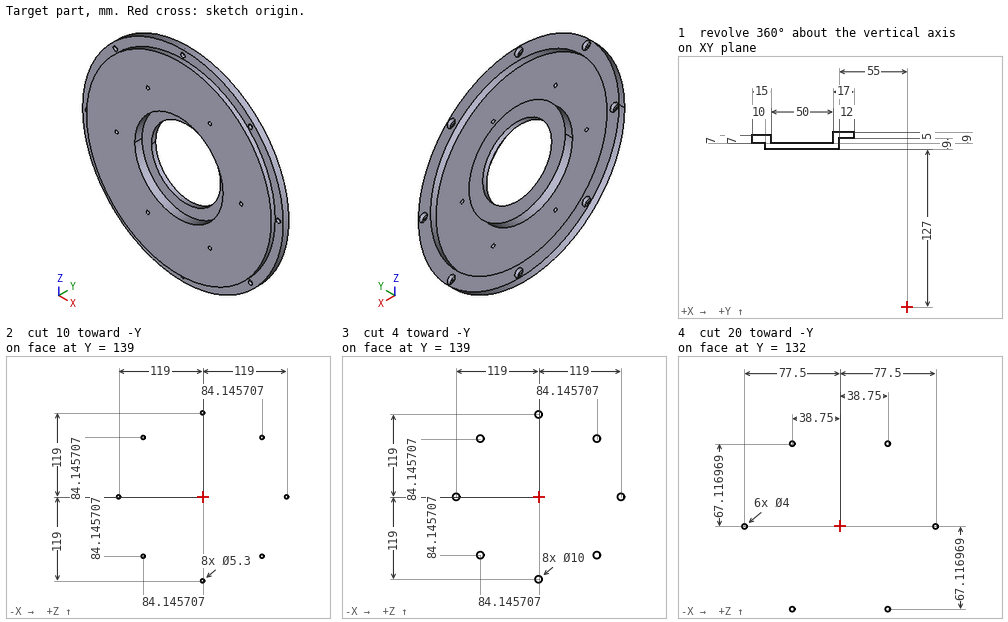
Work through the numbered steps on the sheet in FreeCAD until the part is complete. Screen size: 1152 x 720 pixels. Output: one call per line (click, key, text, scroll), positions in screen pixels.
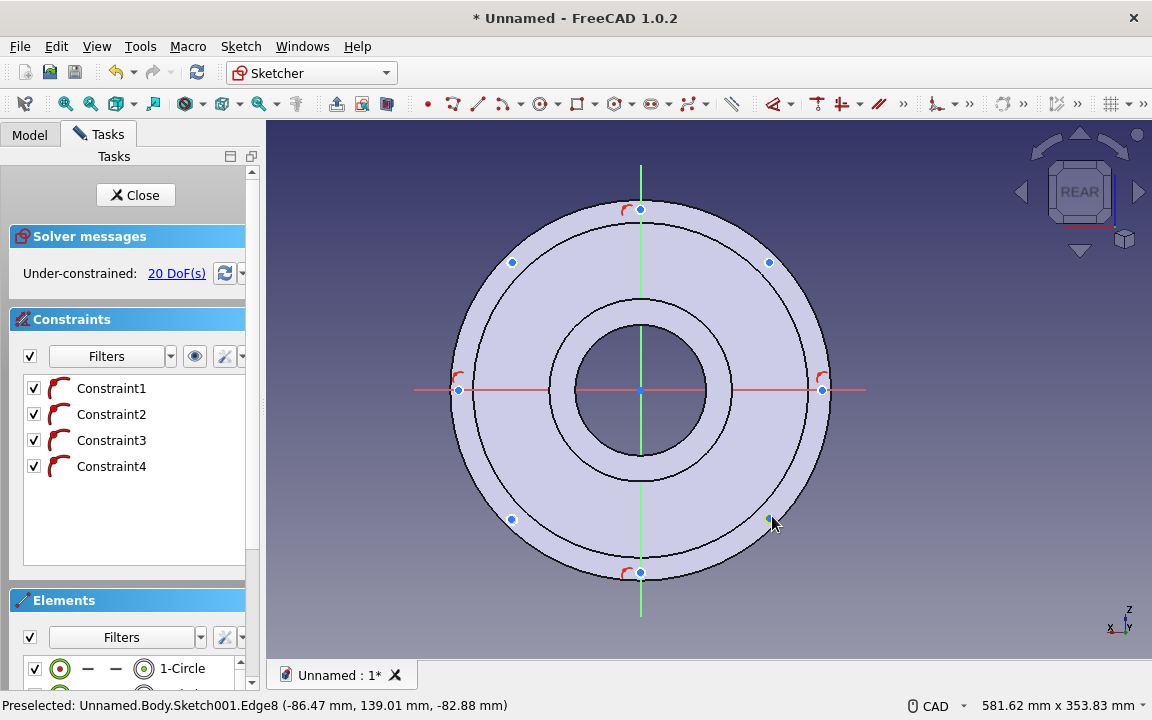
scroll(644, 570, up, 8)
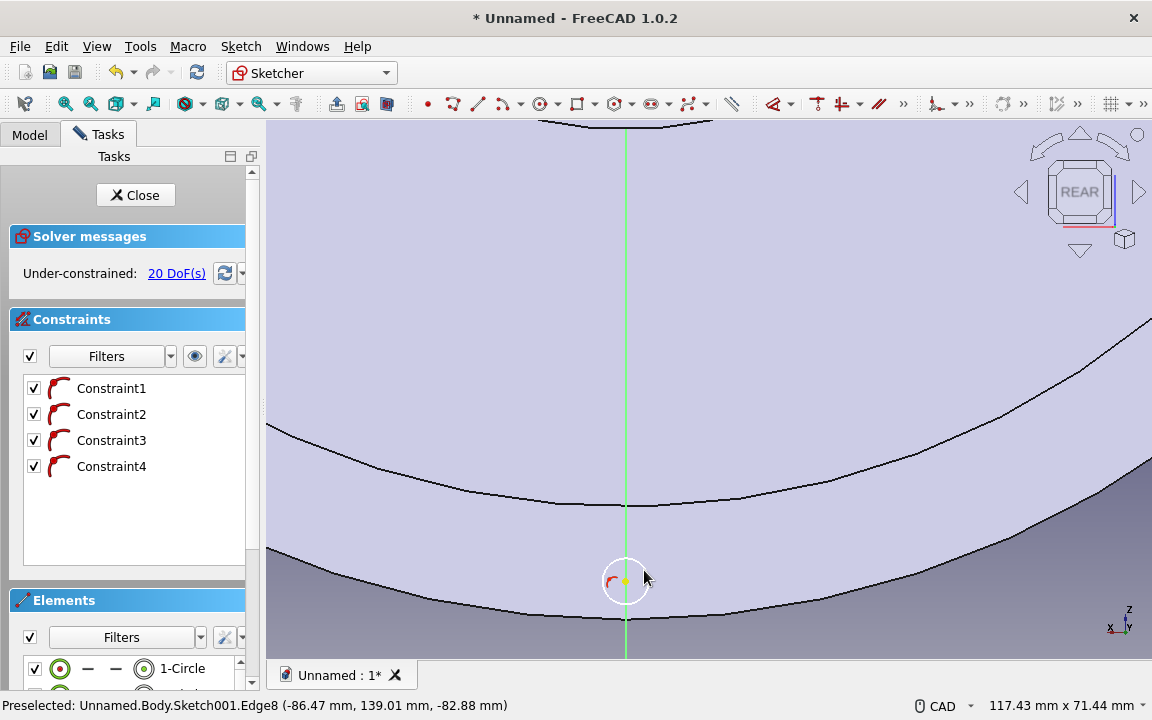
click(642, 565)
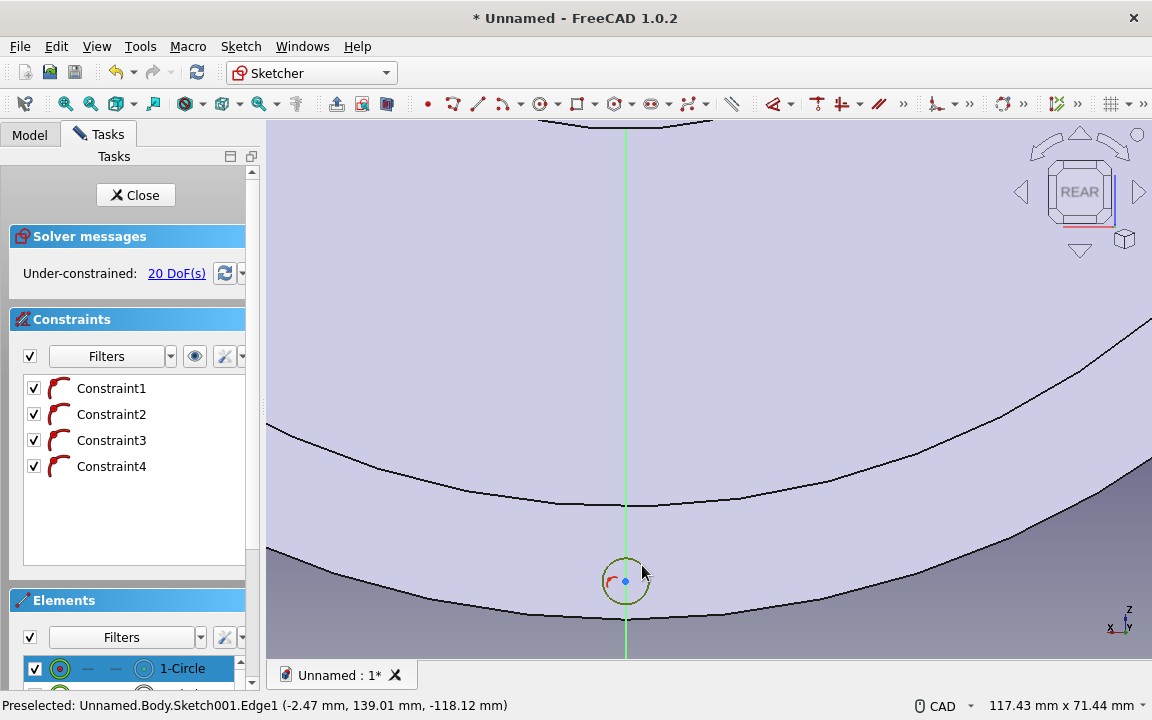
scroll(644, 570, down, 8)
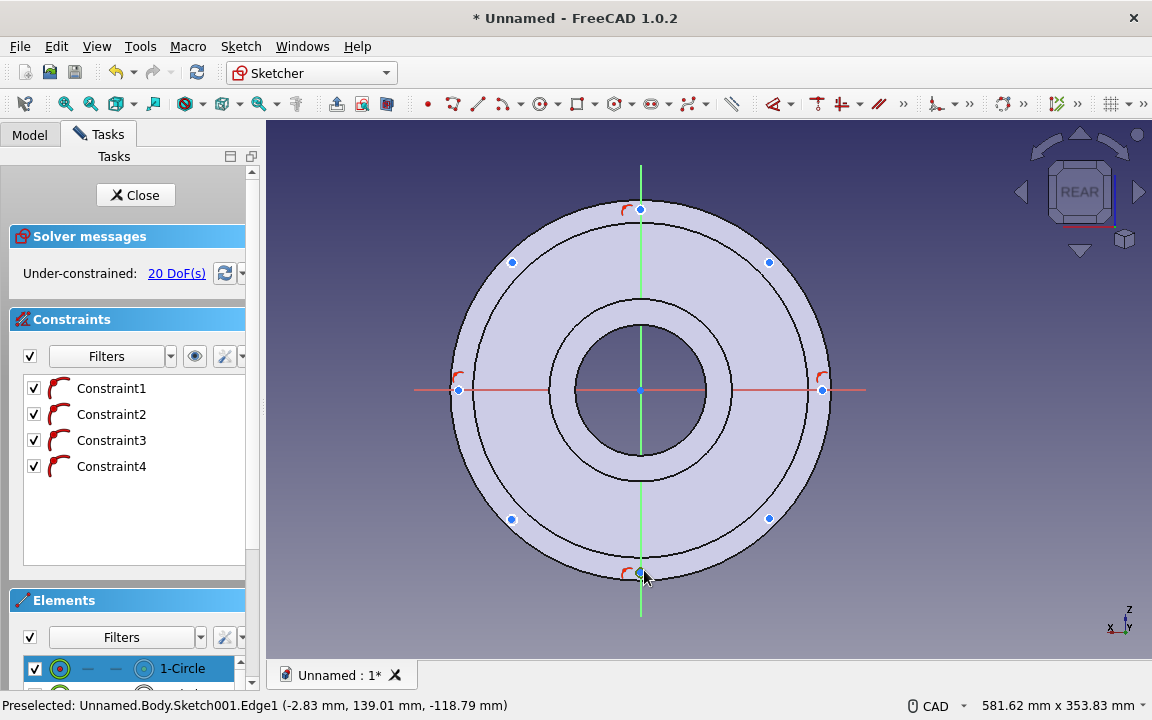
scroll(516, 516, up, 5)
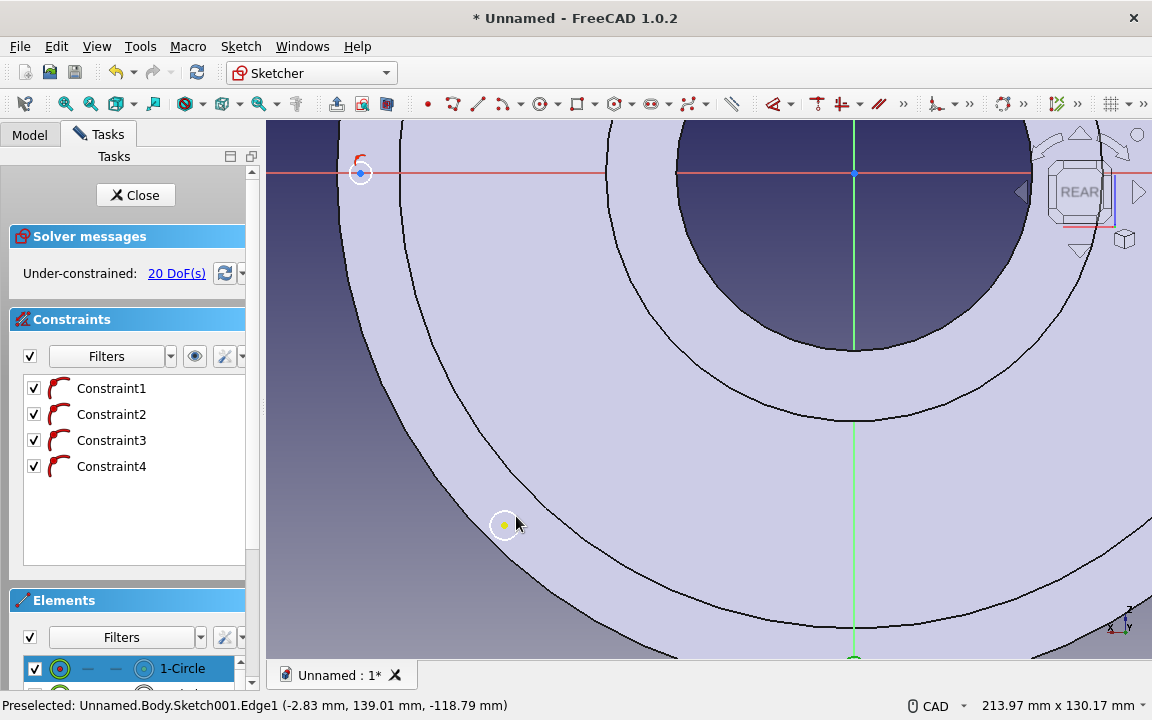
click(515, 515)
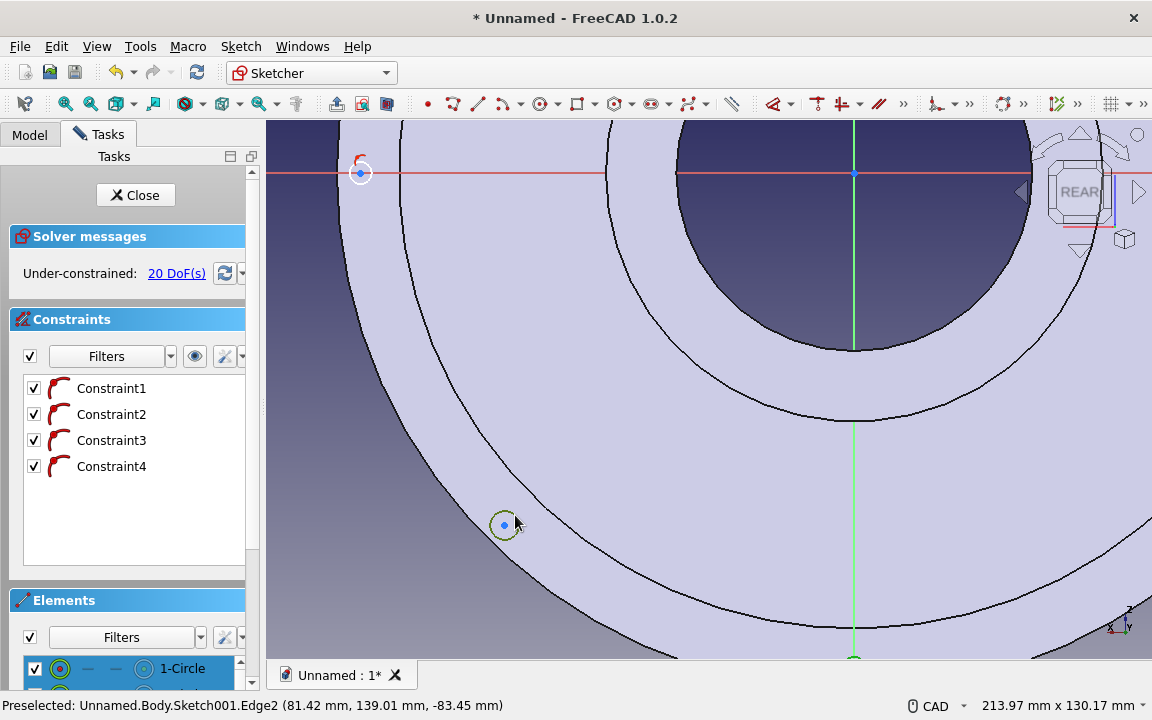
scroll(361, 162, up, 2)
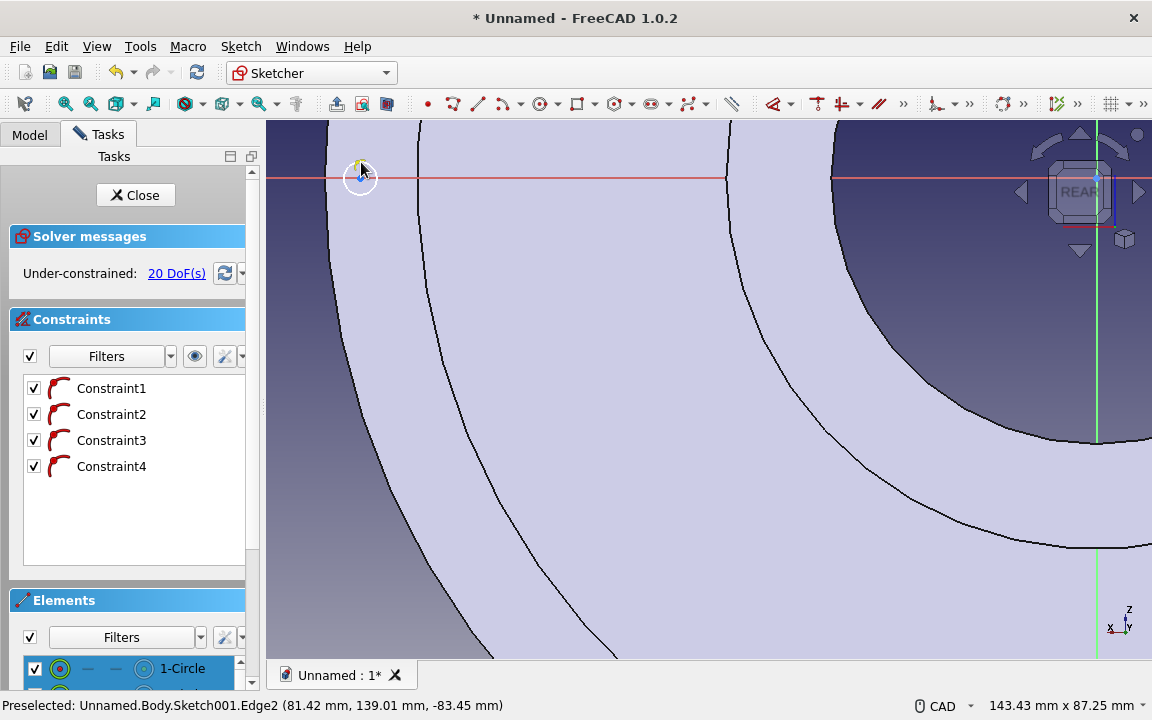
click(344, 178)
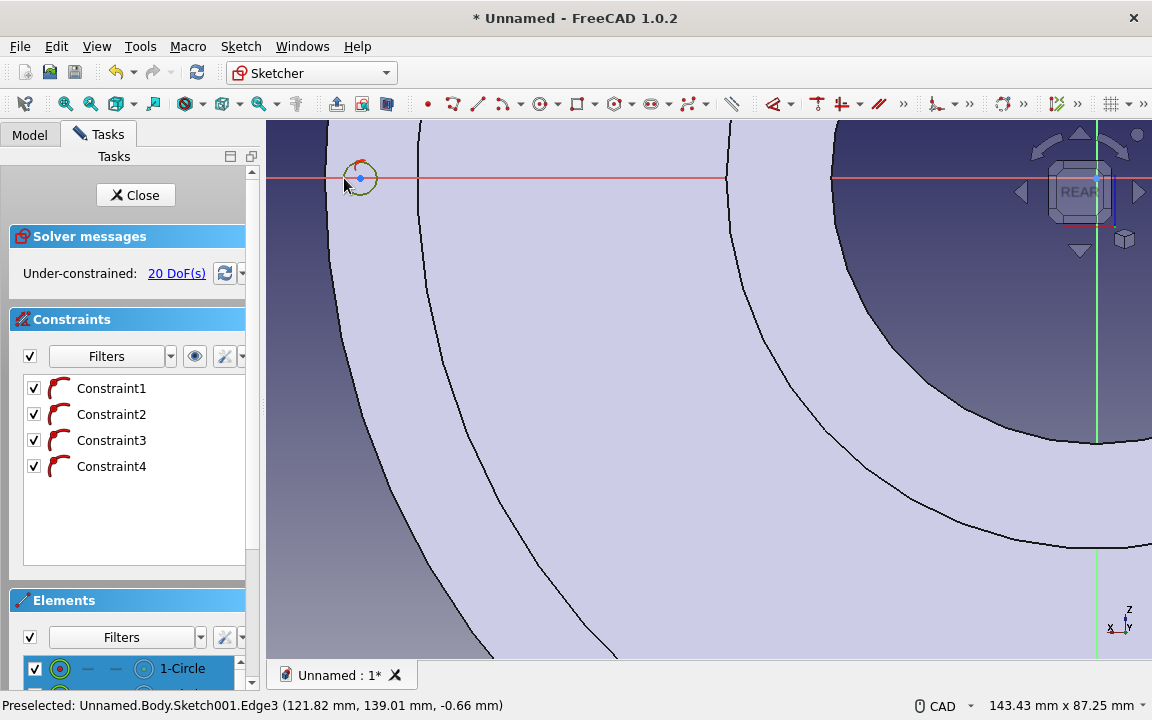
scroll(491, 459, down, 7)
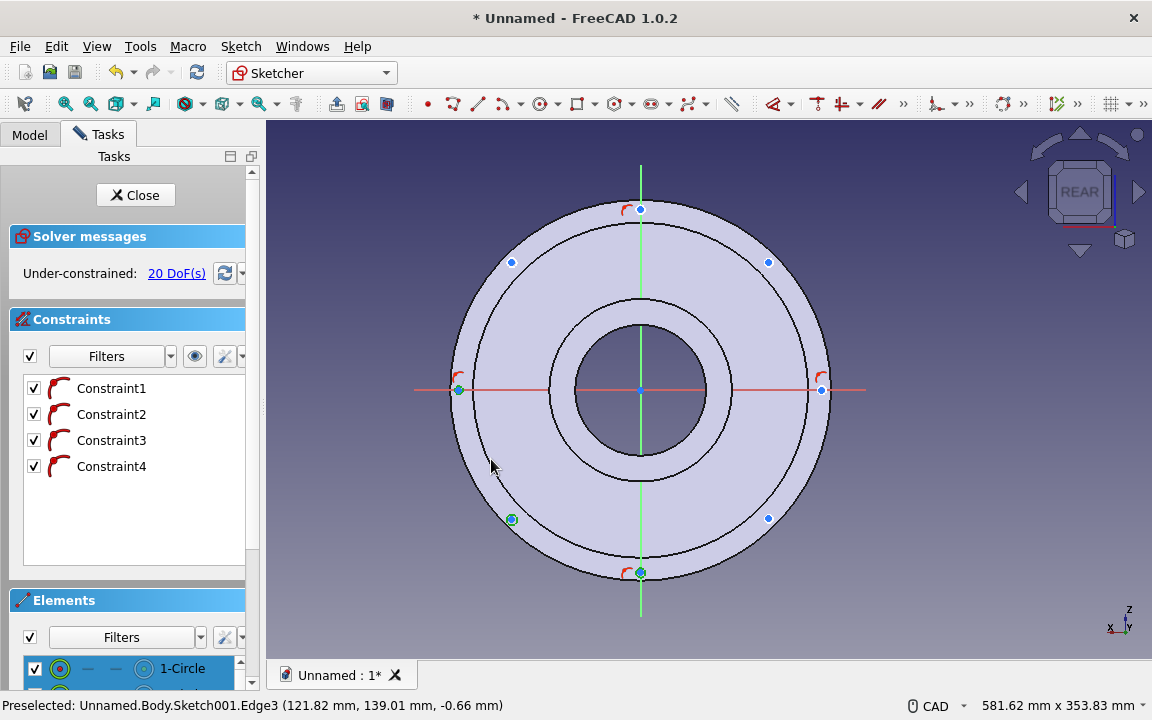
scroll(515, 260, up, 6)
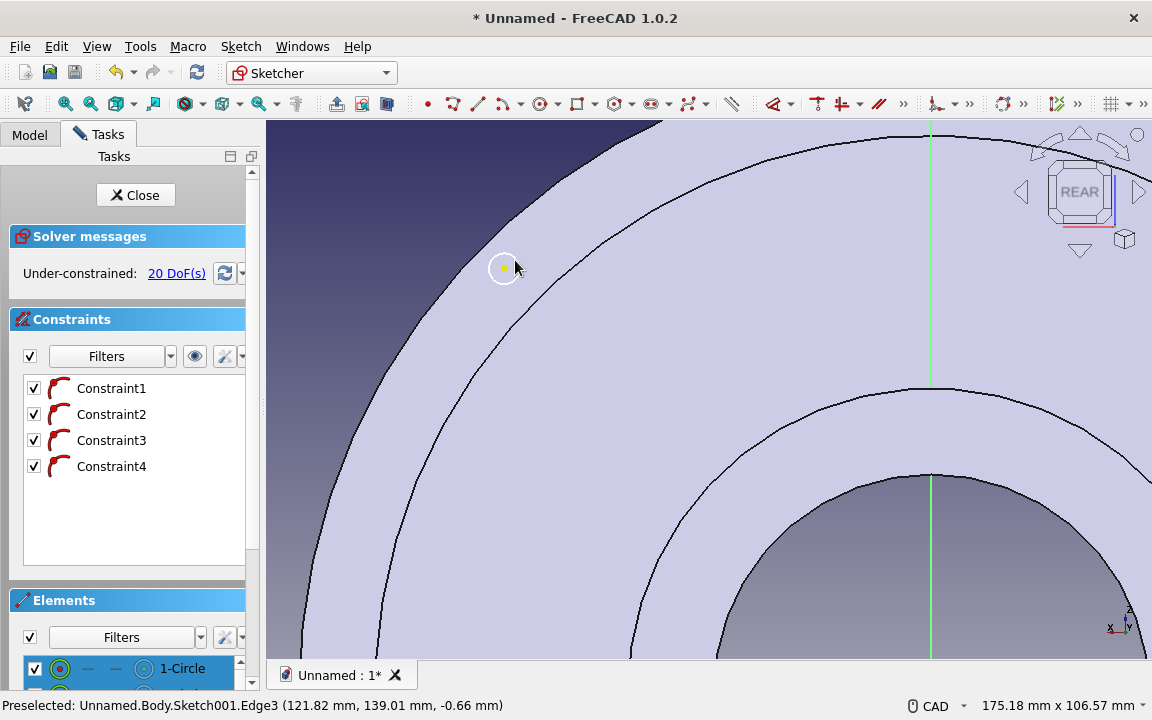
click(515, 258)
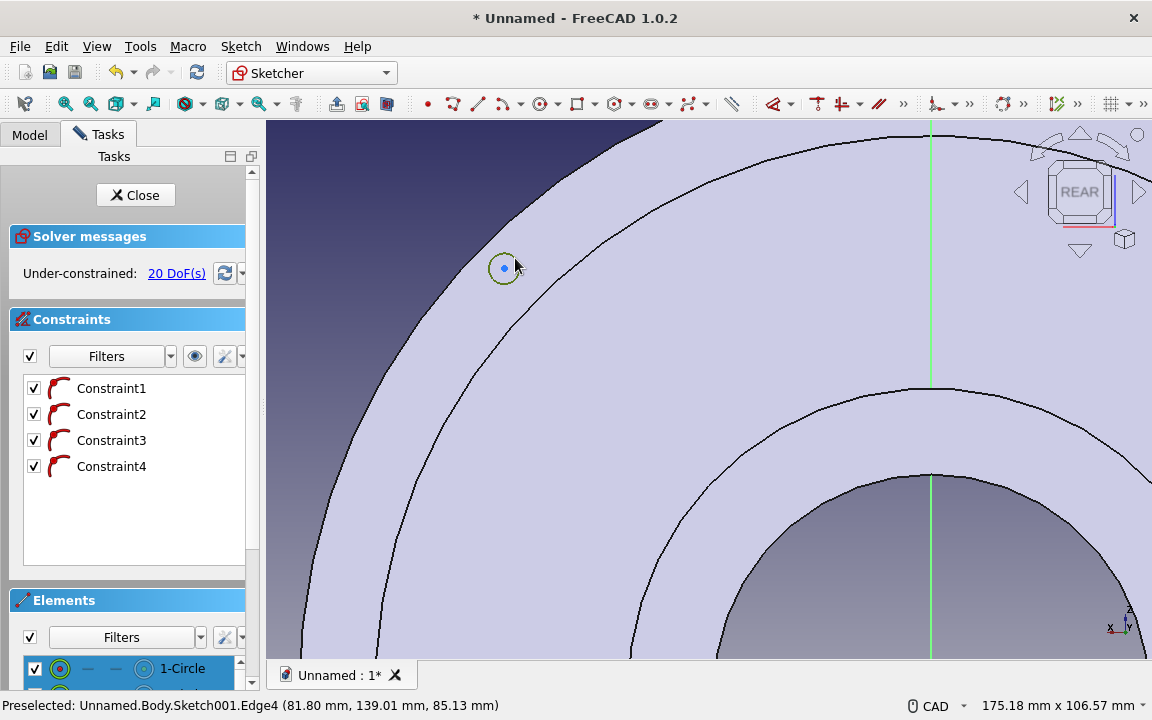
scroll(515, 259, down, 6)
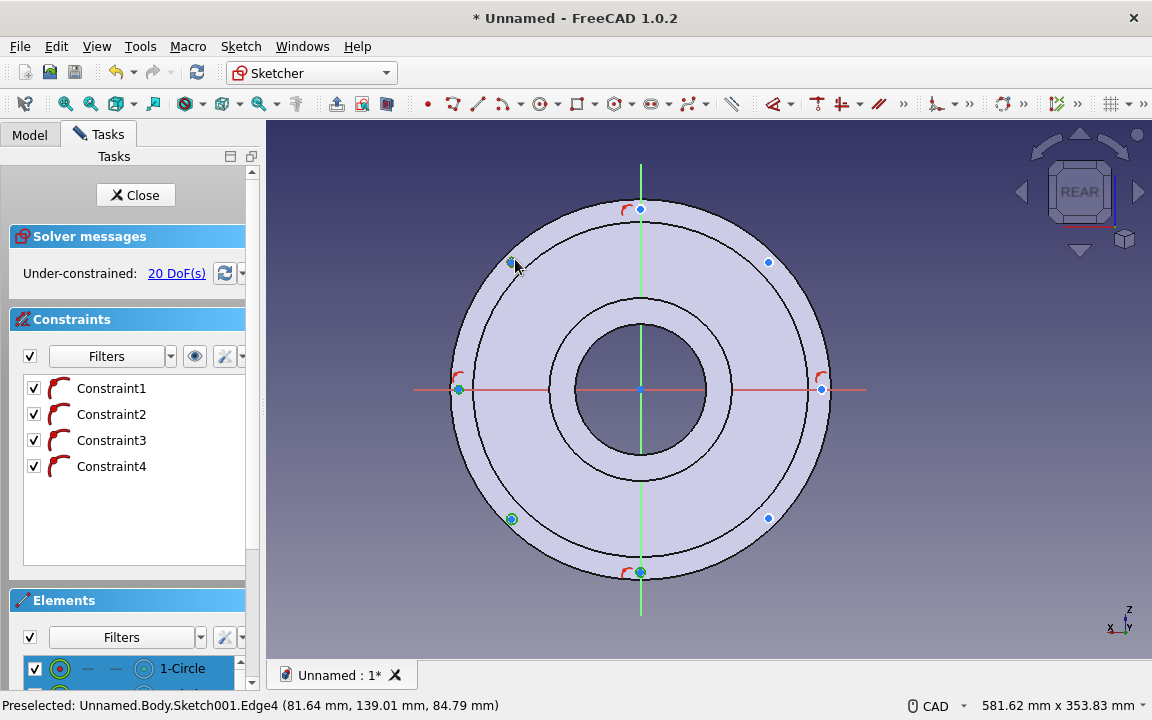
scroll(644, 206, up, 8)